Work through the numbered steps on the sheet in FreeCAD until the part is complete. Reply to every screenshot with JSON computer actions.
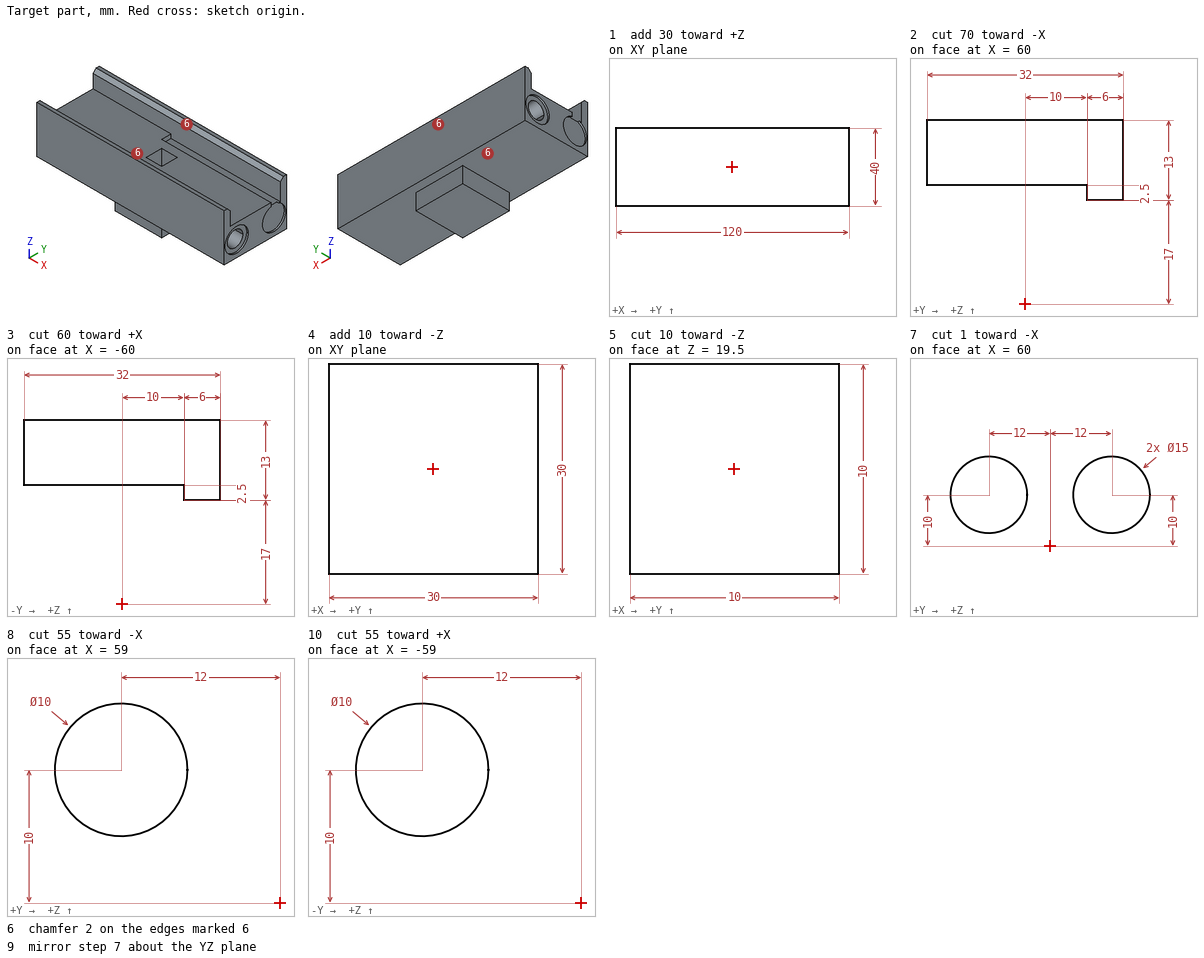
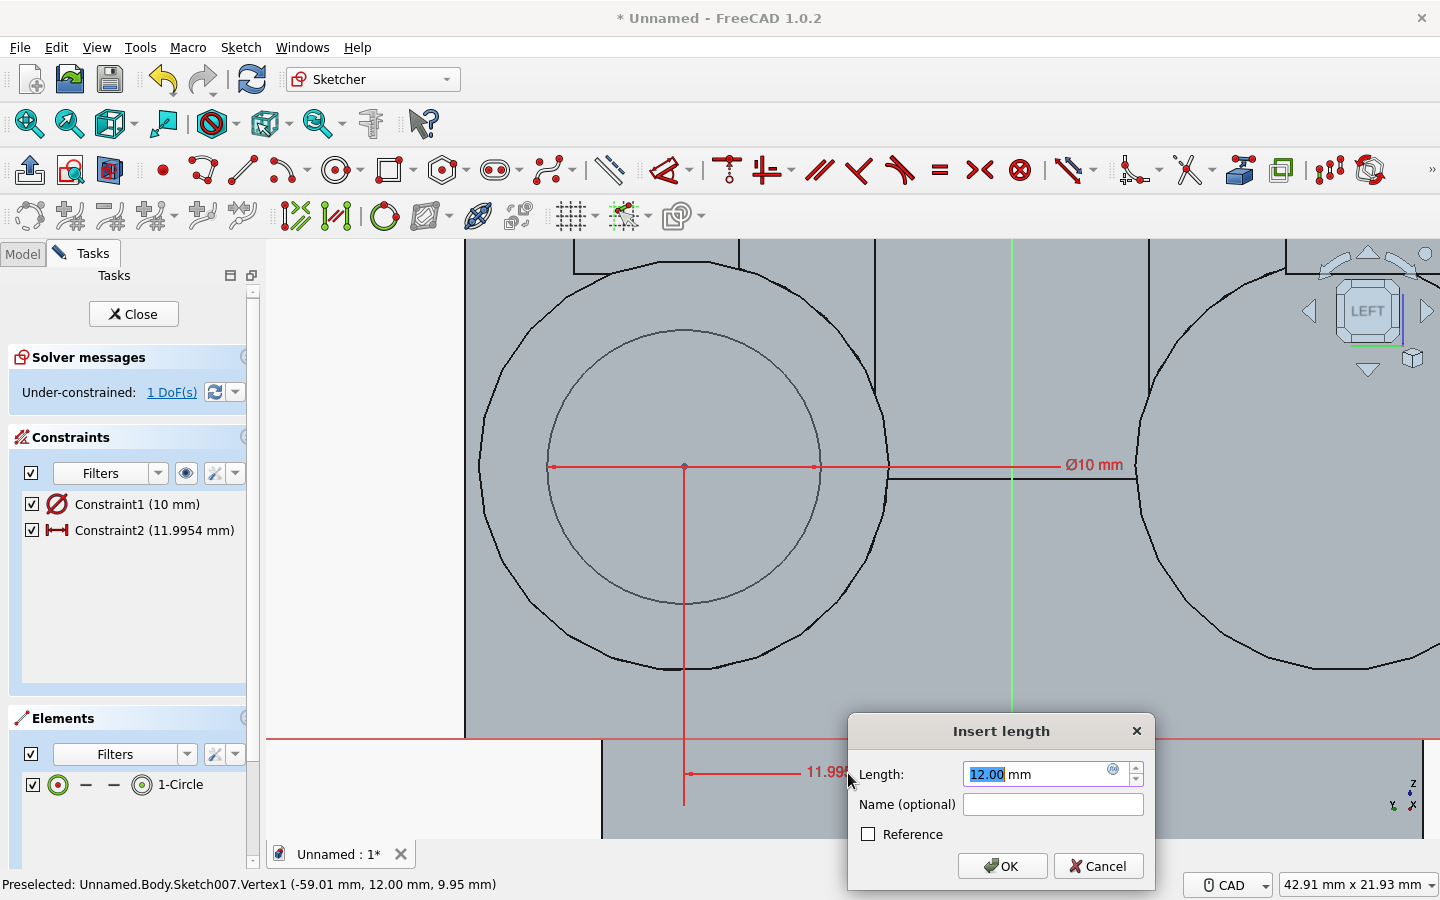
{"action": "type", "text": "12"}
{"action": "key", "text": "Return"}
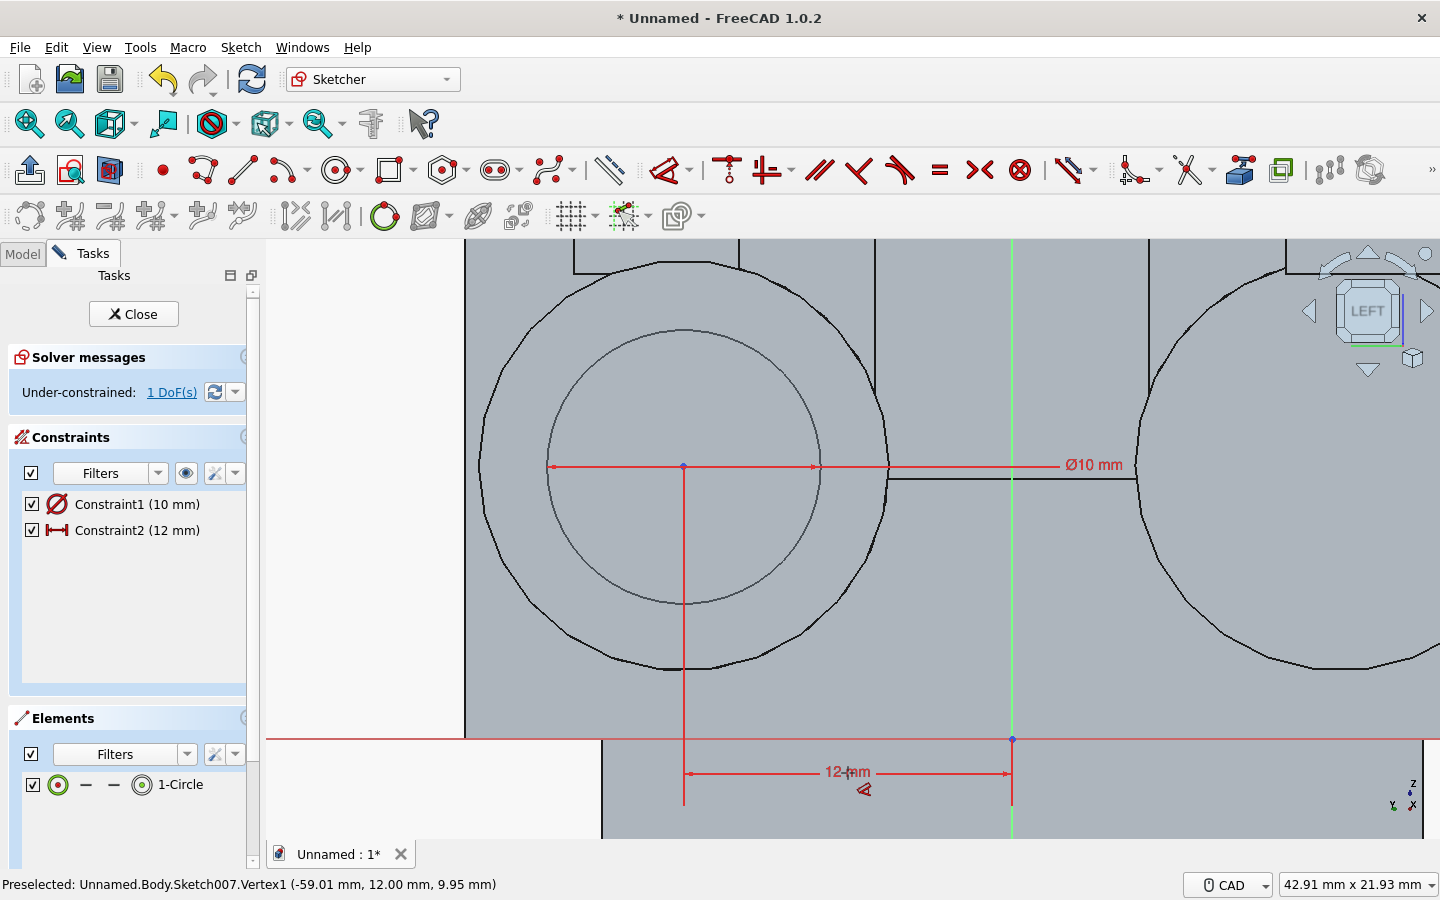
{"action": "left_click", "coordinate": [684, 467]}
{"action": "left_click", "coordinate": [1046, 603]}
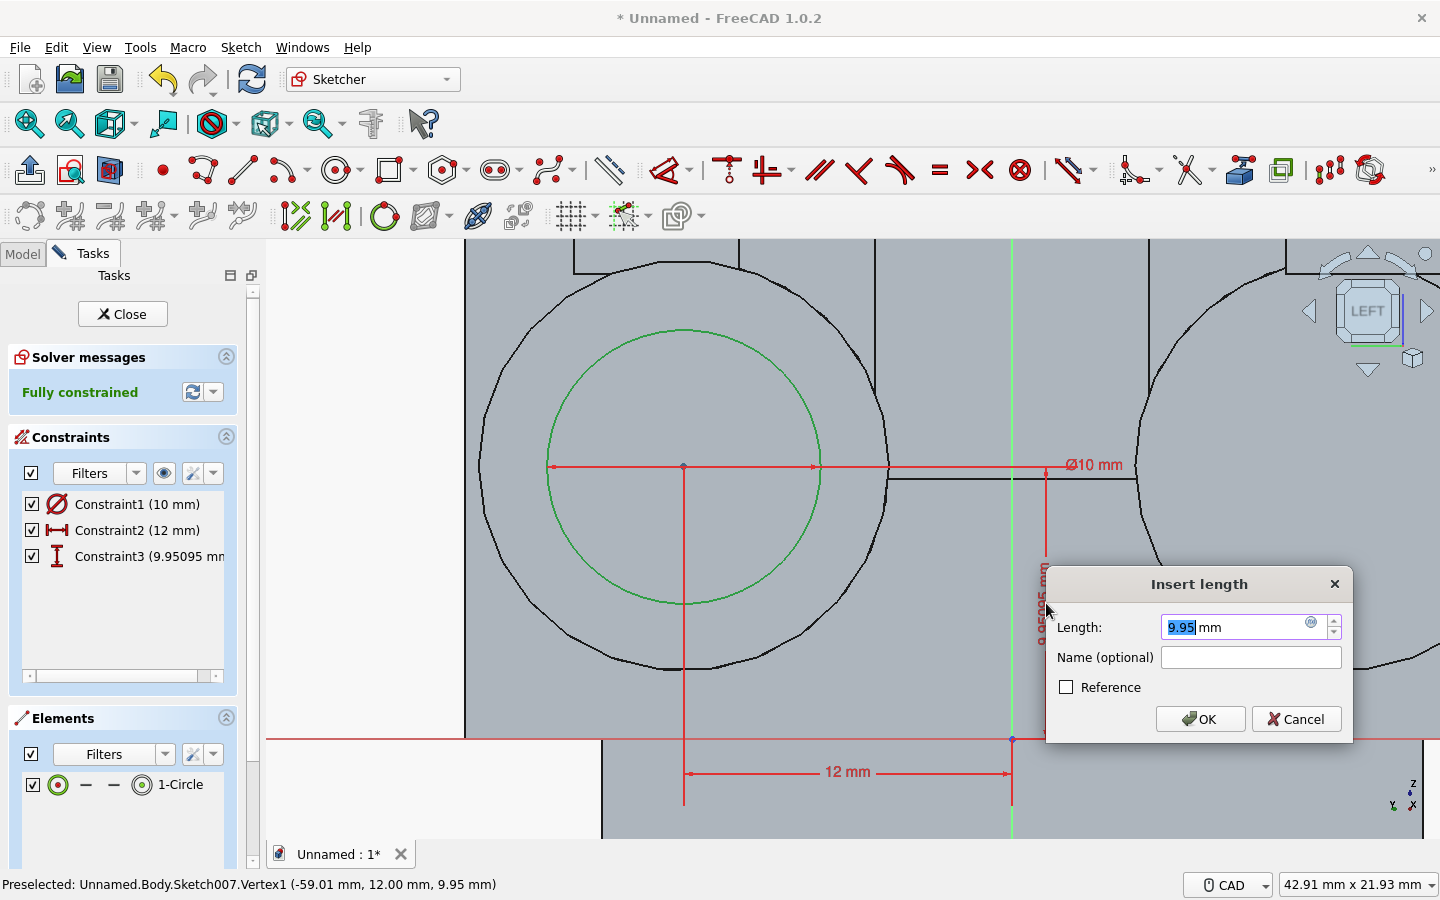
{"action": "type", "text": "10"}
{"action": "key", "text": "Return"}
{"action": "key", "text": "Escape"}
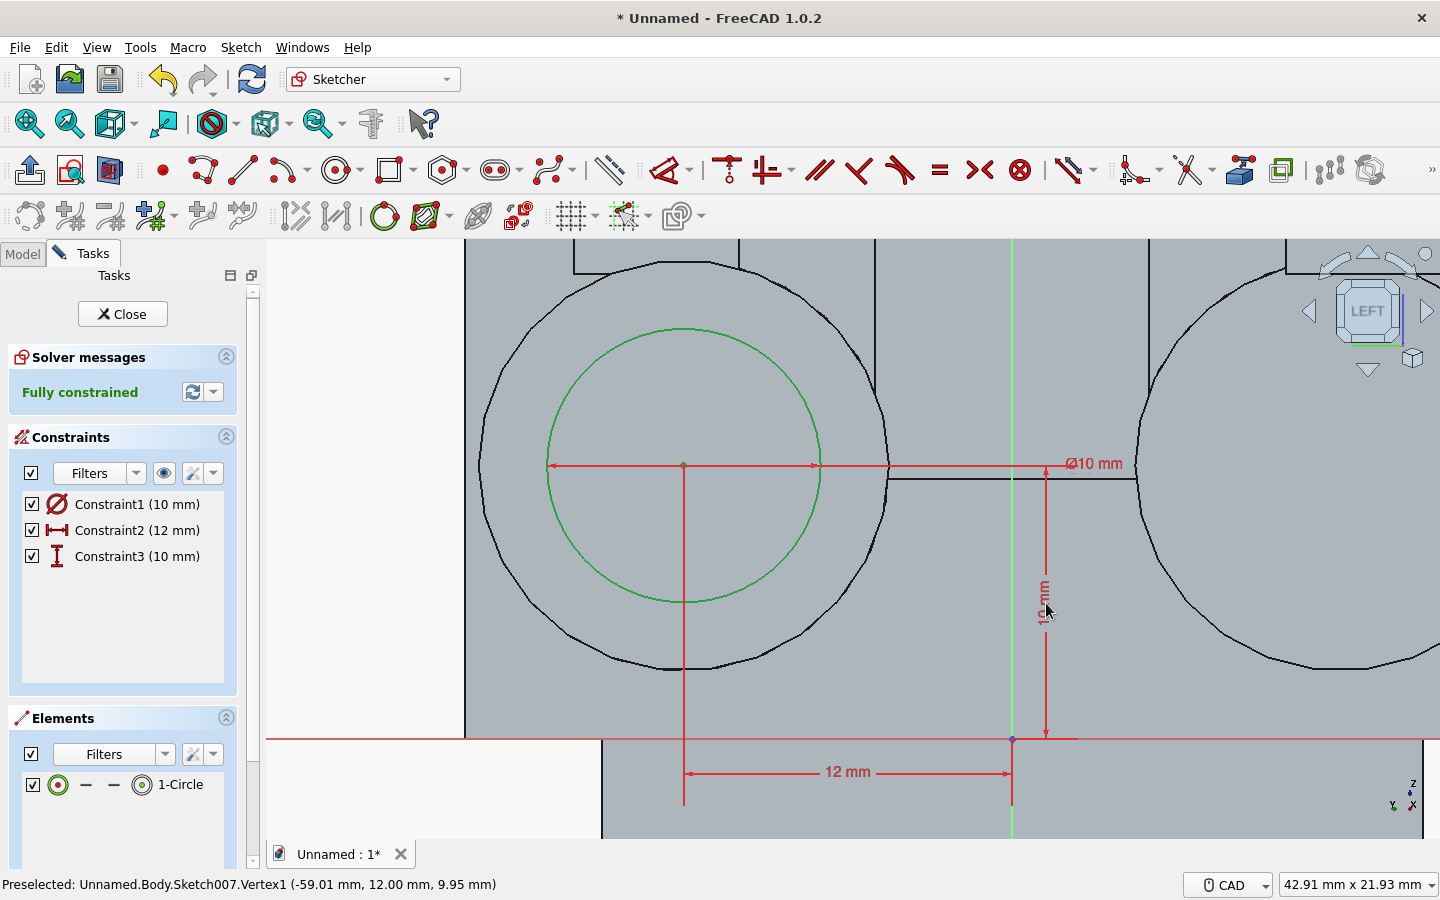
{"action": "left_click", "coordinate": [123, 314]}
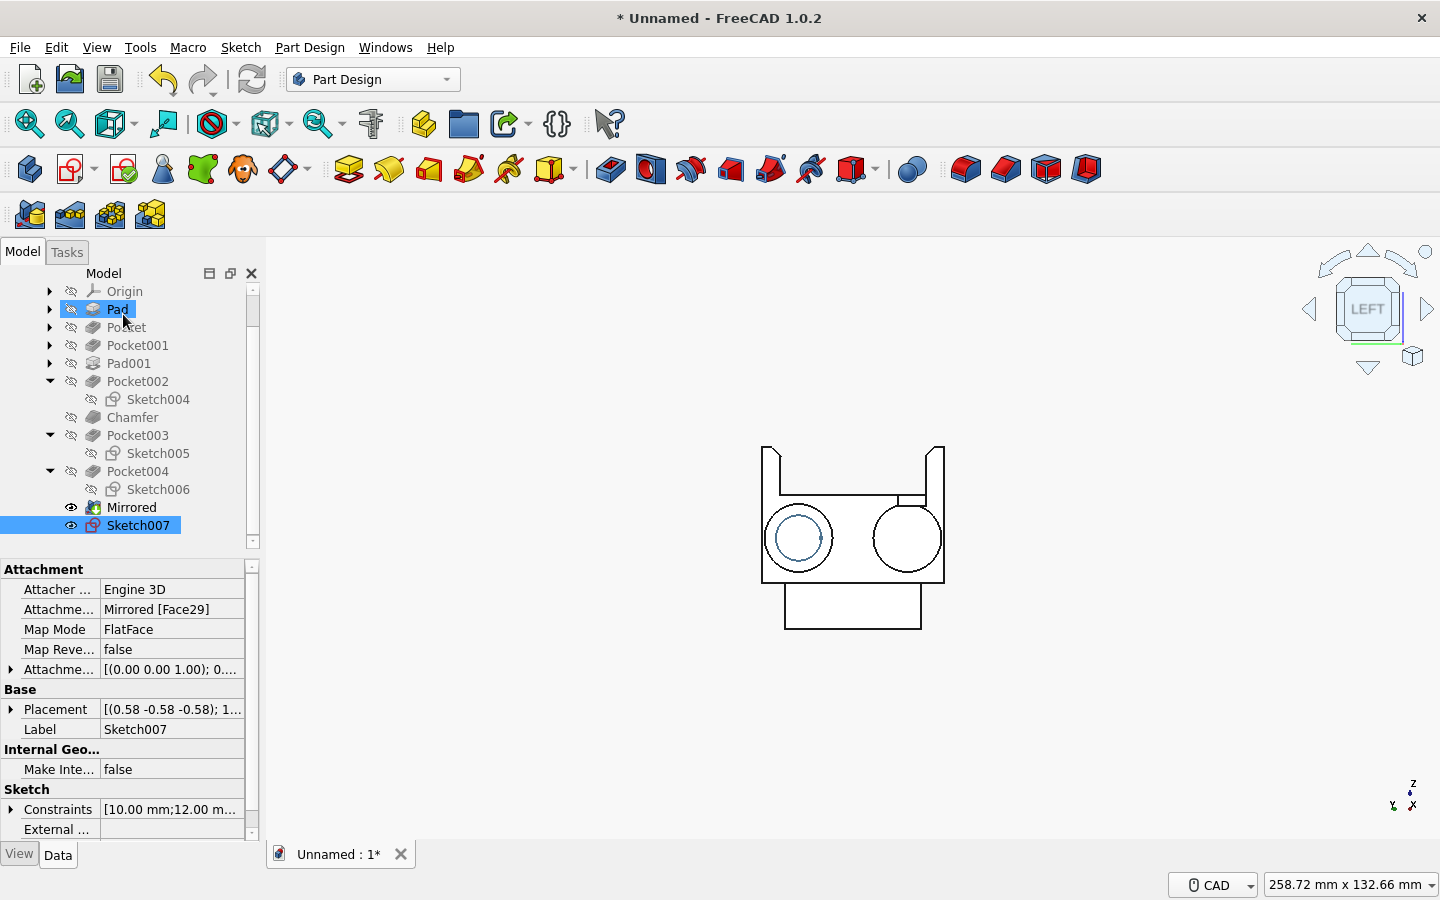
{"action": "left_click", "coordinate": [612, 170]}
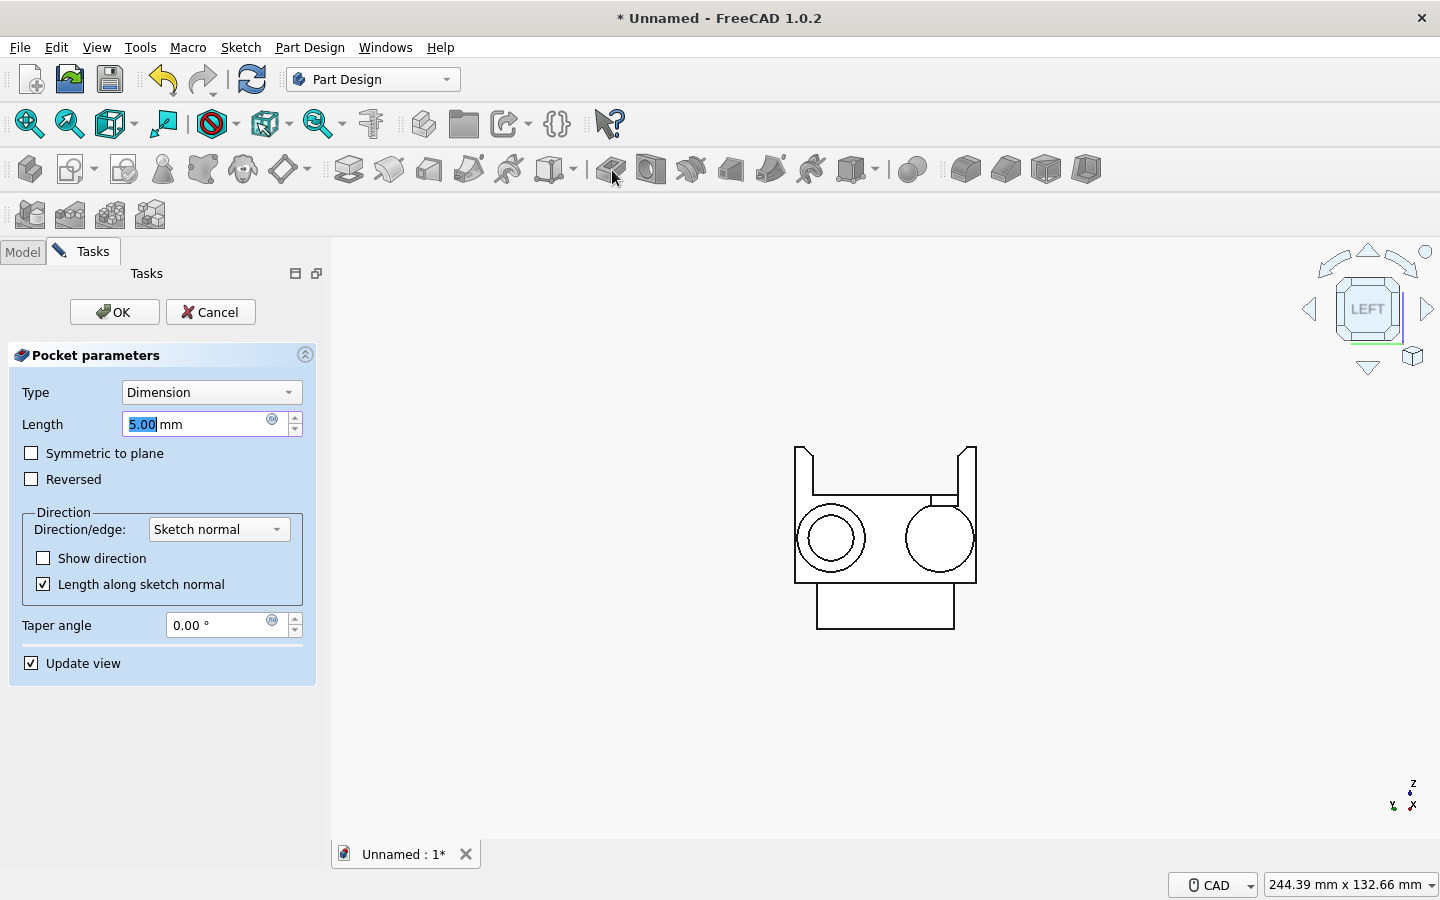
{"action": "type", "text": "55"}
{"action": "key", "text": "Tab"}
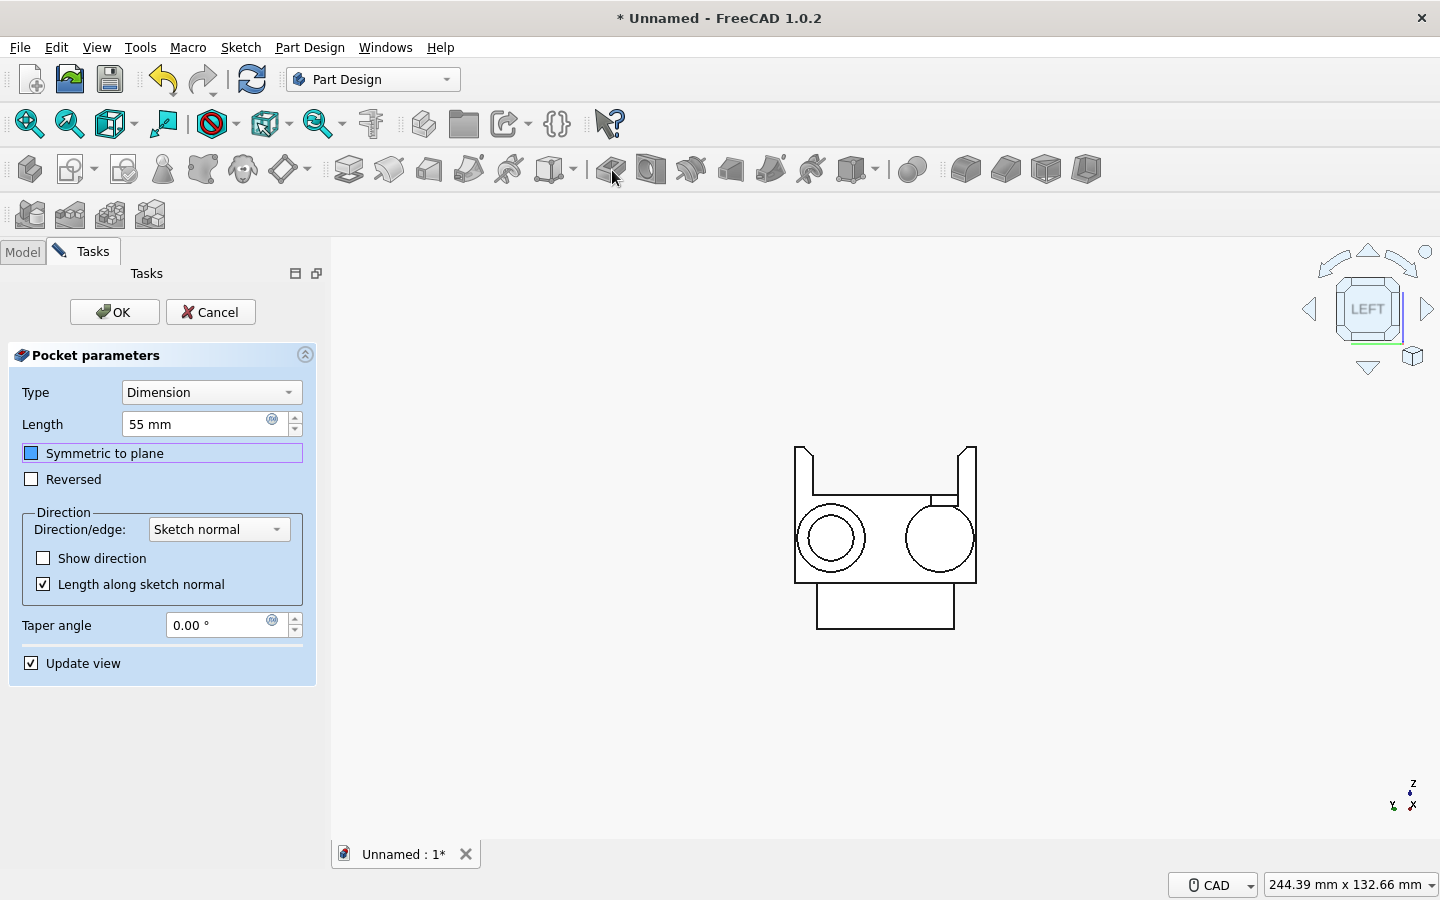
{"action": "left_click", "coordinate": [115, 312]}